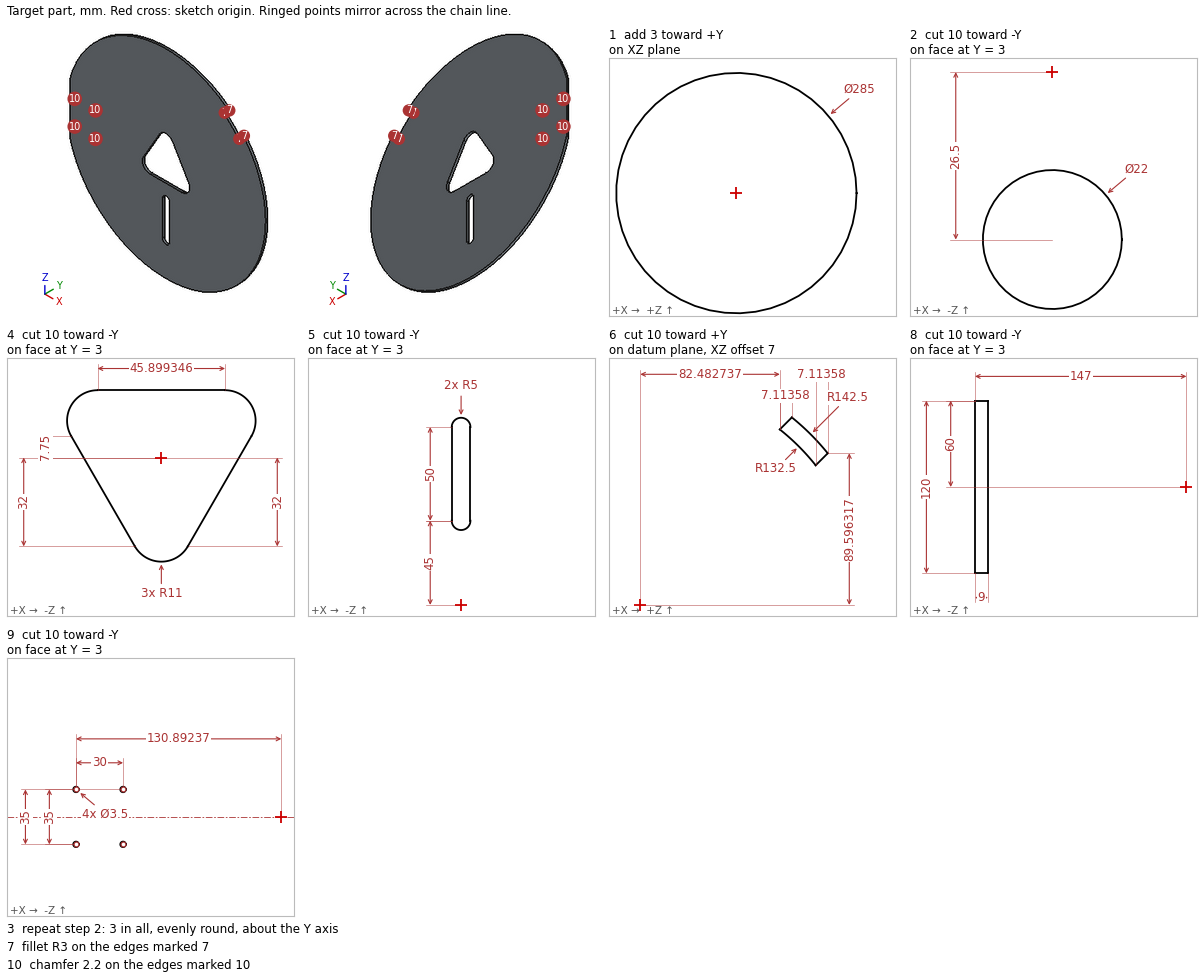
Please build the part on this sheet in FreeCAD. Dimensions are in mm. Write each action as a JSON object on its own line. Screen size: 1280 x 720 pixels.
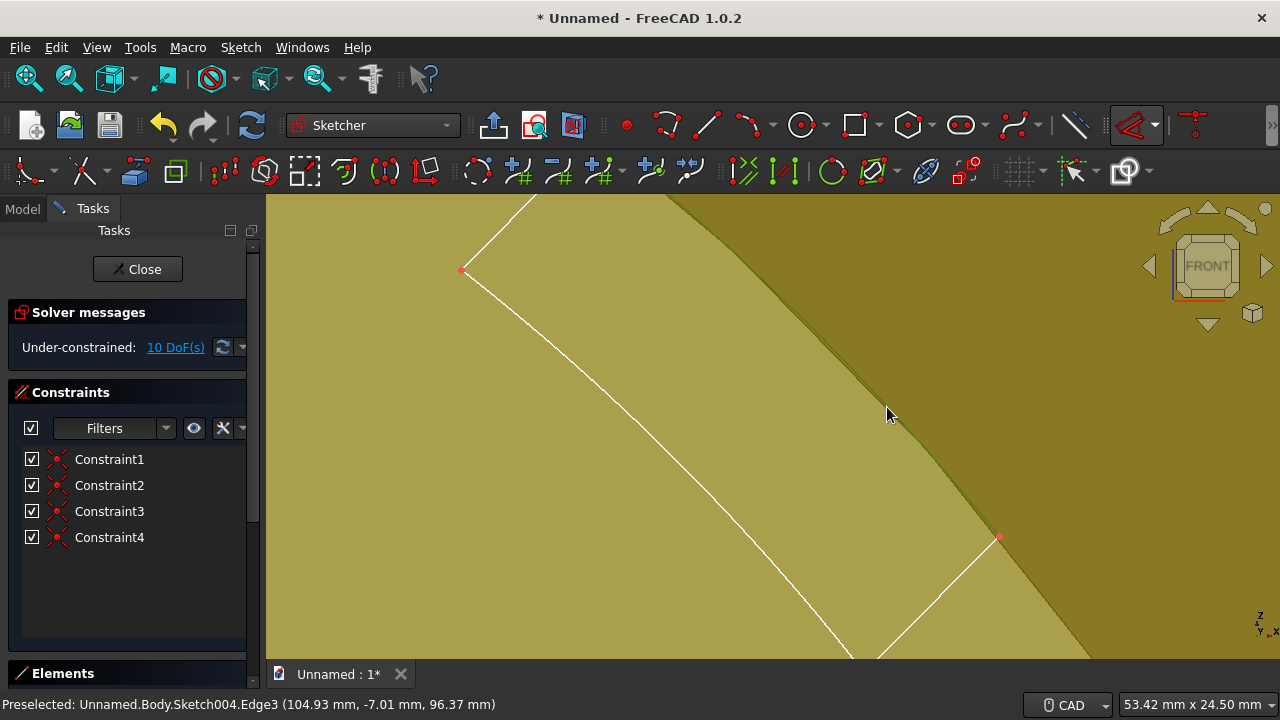
{"action": "left_click", "coordinate": [754, 542]}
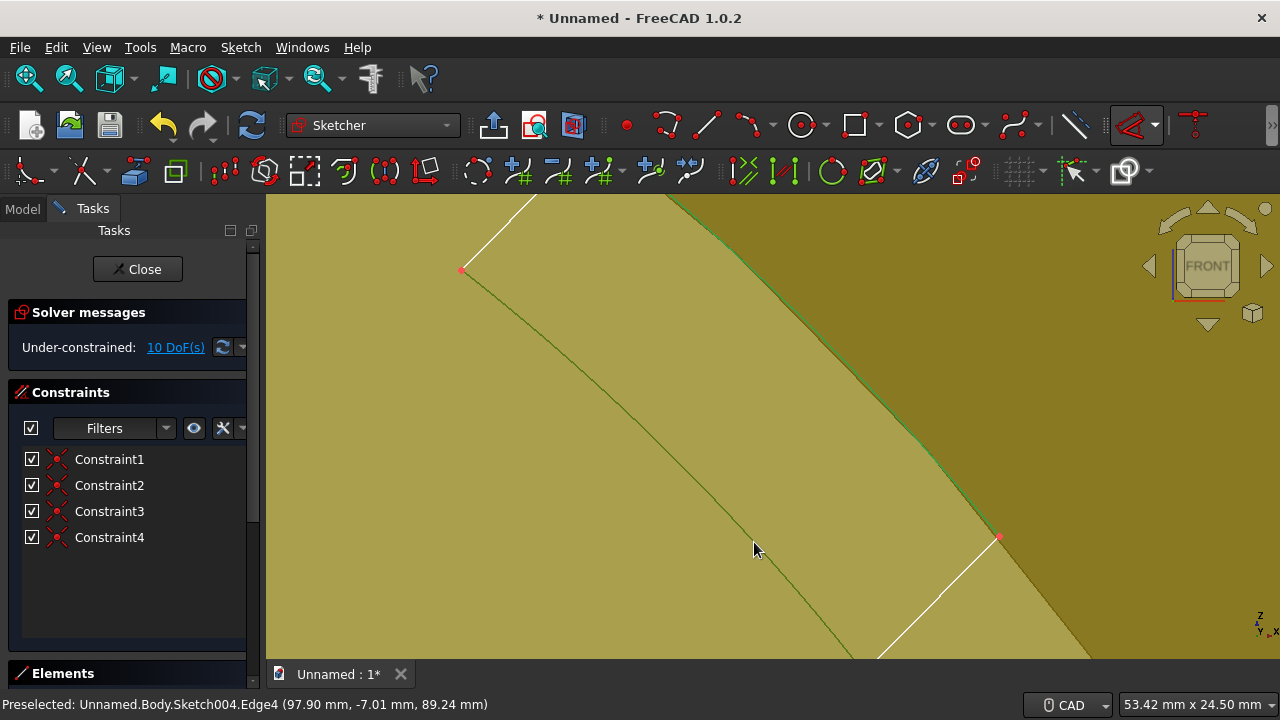
{"action": "left_click", "coordinate": [1194, 126]}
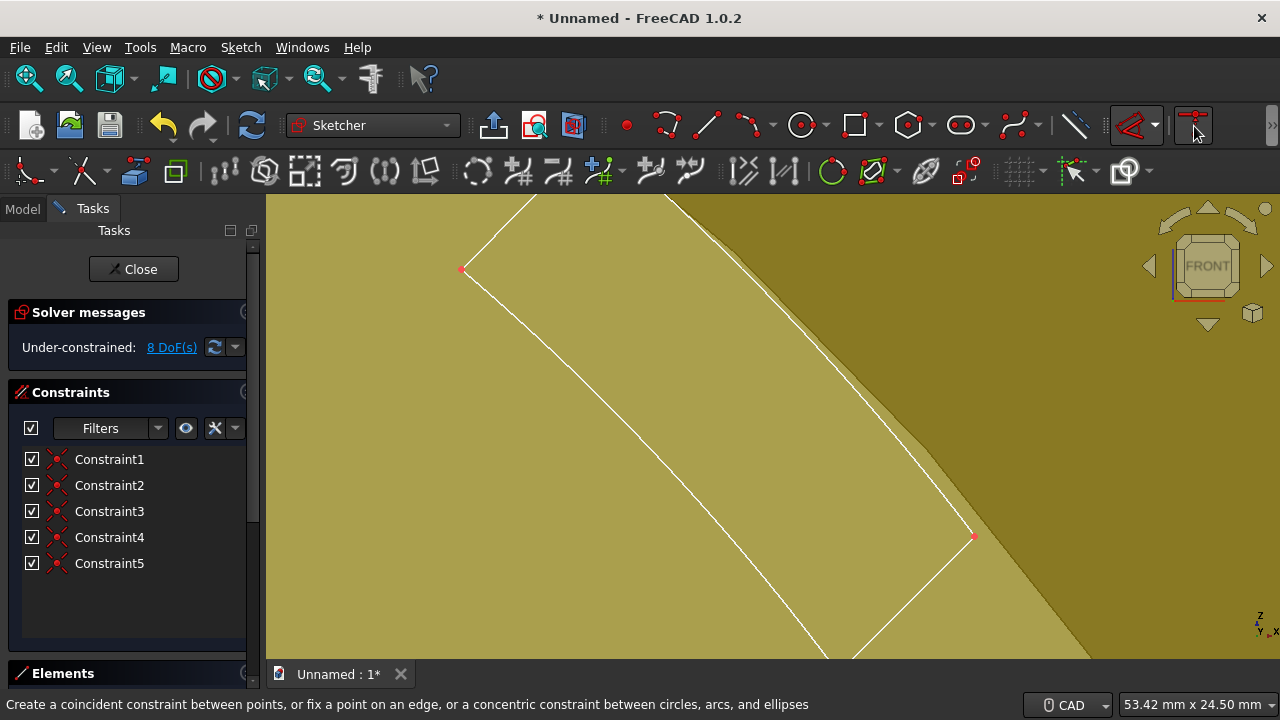
{"action": "scroll", "coordinate": [673, 457], "scroll_direction": "down", "scroll_amount": 3}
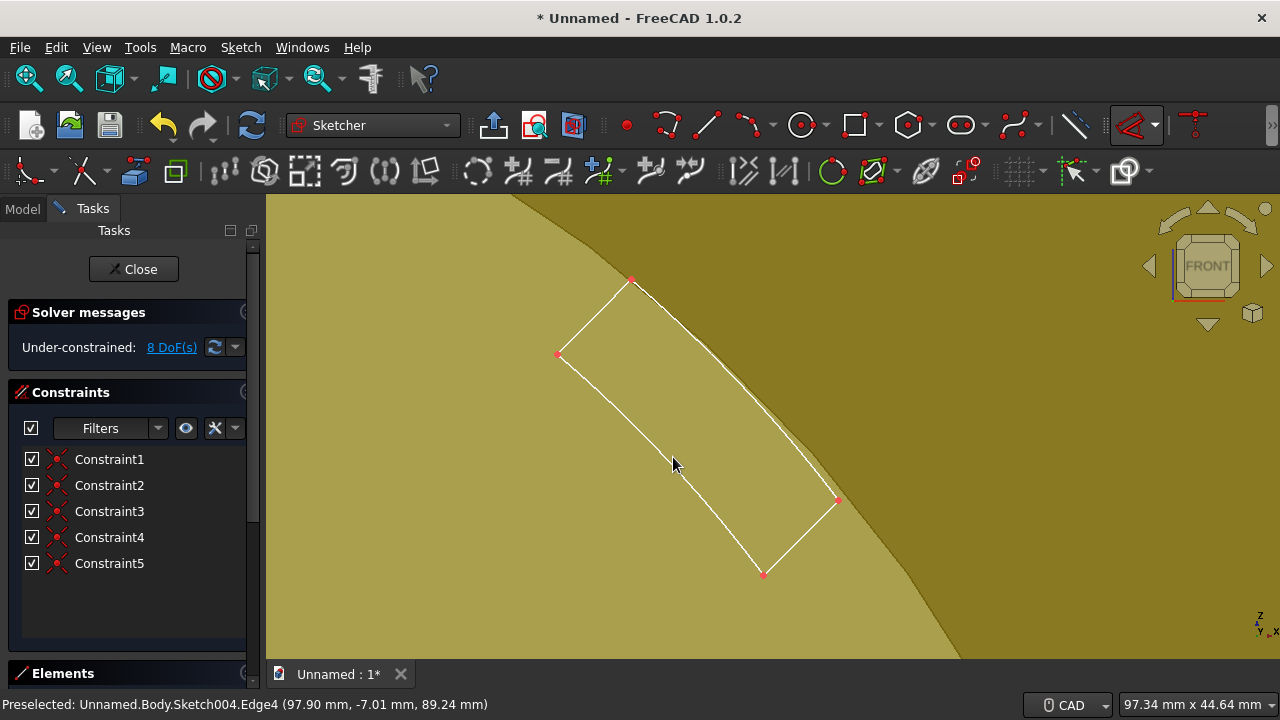
{"action": "scroll", "coordinate": [846, 291], "scroll_direction": "down", "scroll_amount": 7}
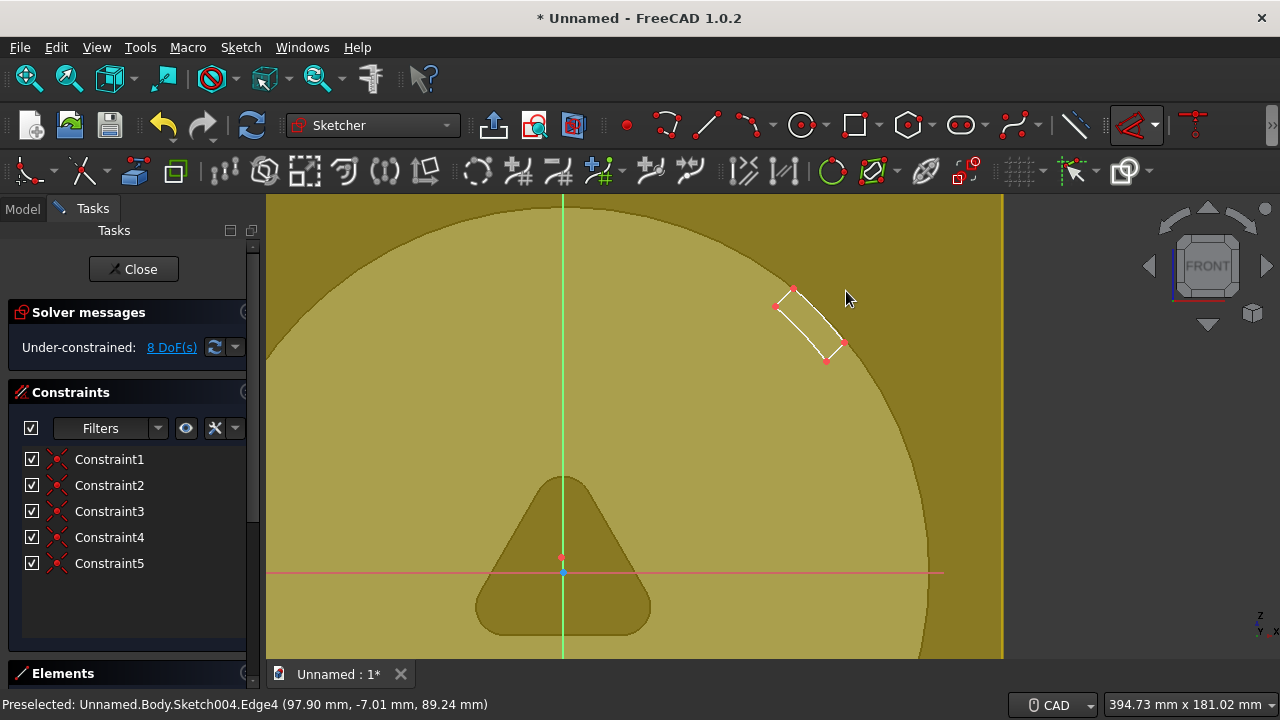
{"action": "left_click_drag", "start_coordinate": [552, 548], "coordinate": [573, 583]}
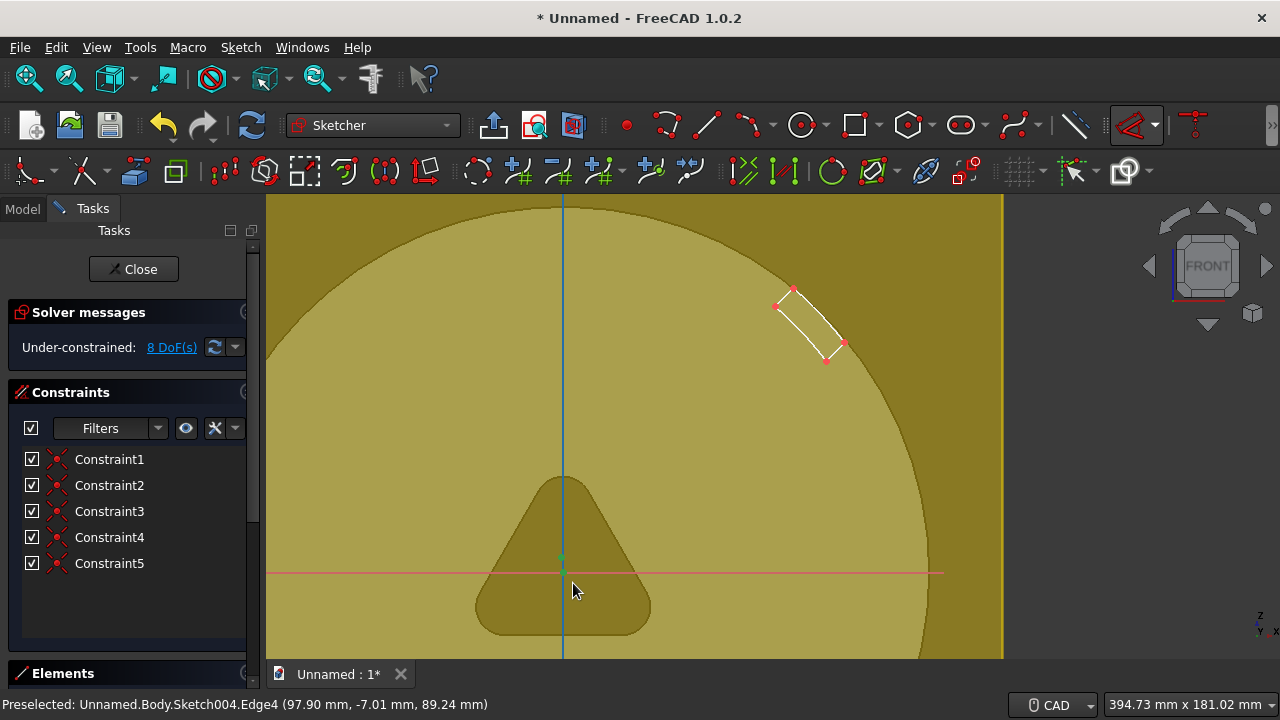
{"action": "left_click", "coordinate": [1194, 126]}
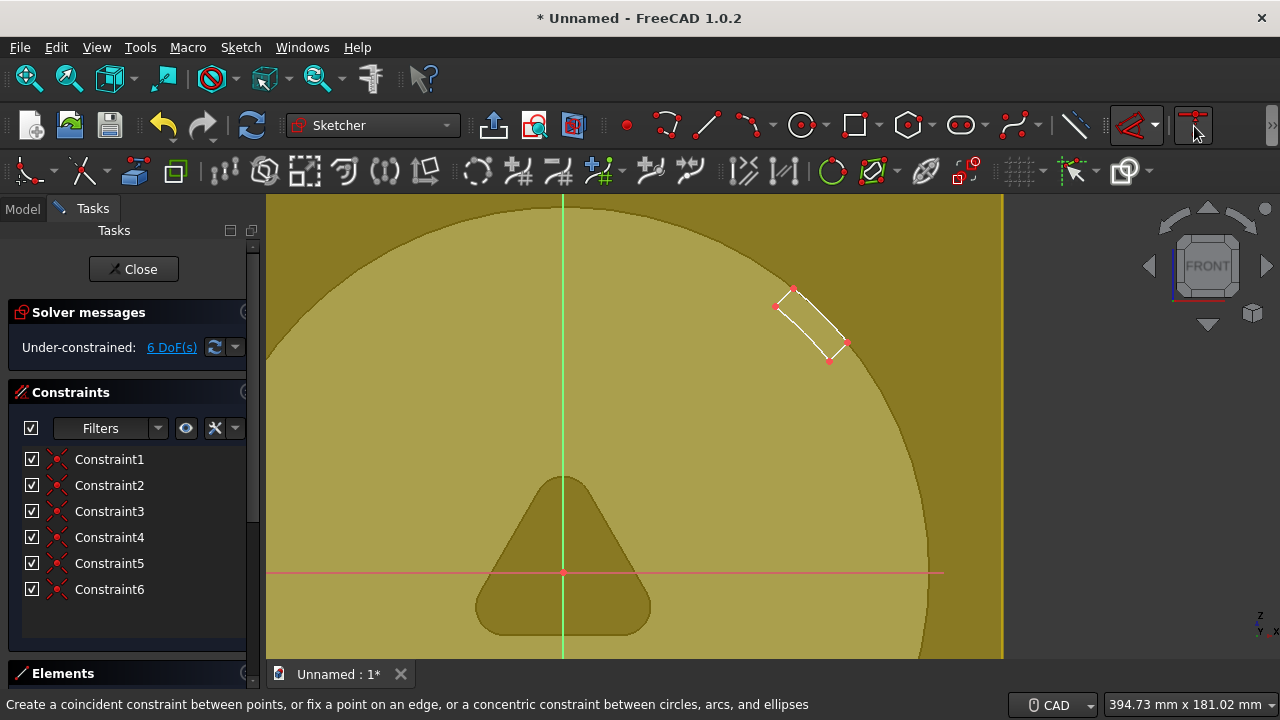
{"action": "left_click", "coordinate": [833, 325]}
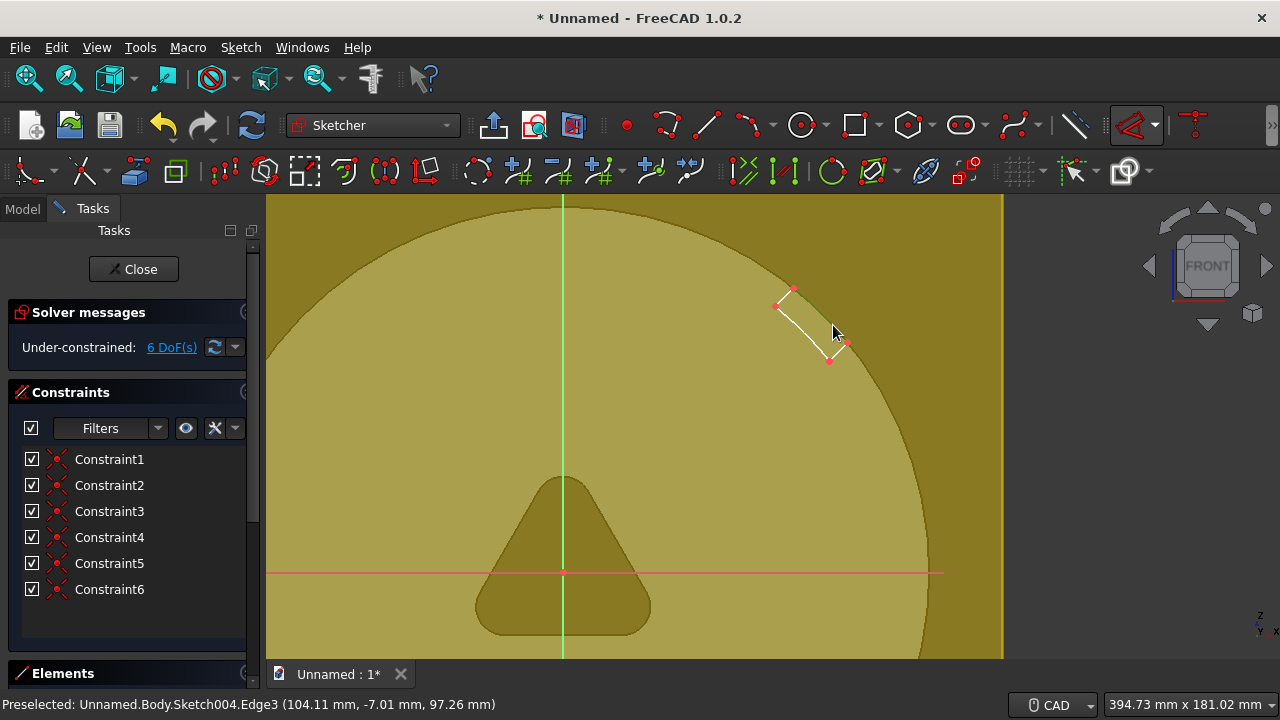
{"action": "left_click", "coordinate": [1158, 126]}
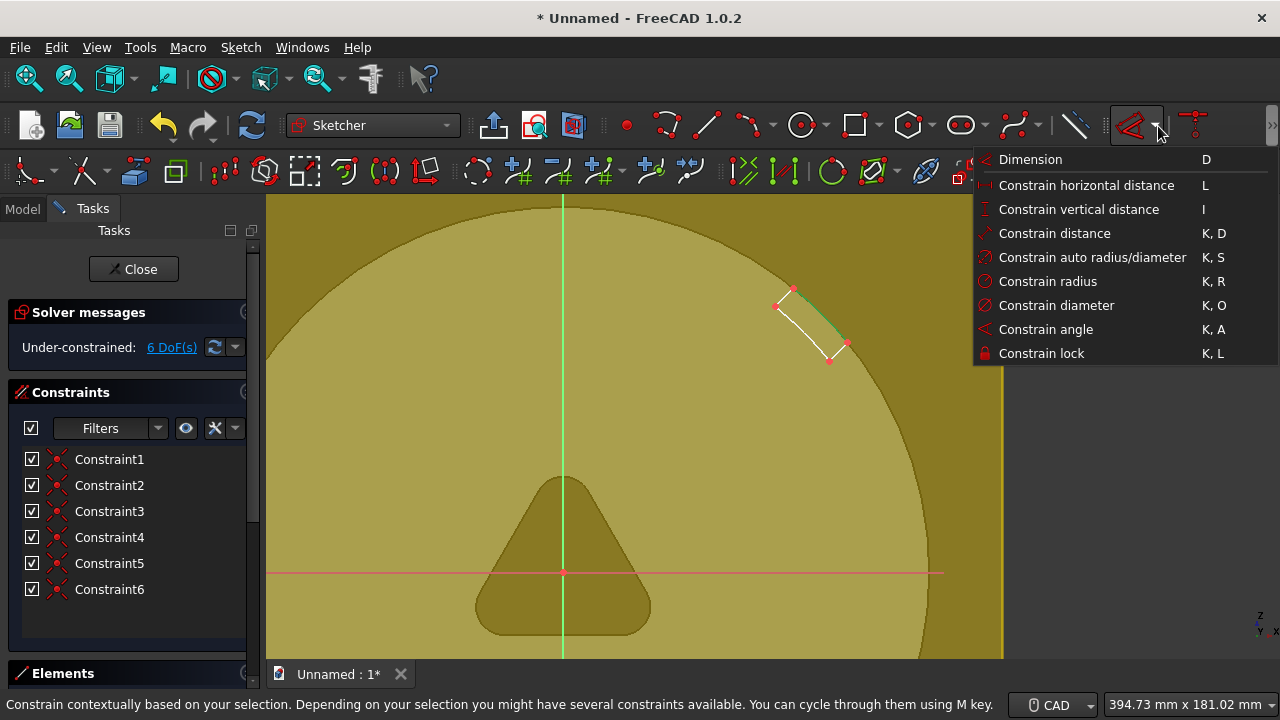
{"action": "left_click", "coordinate": [1126, 281]}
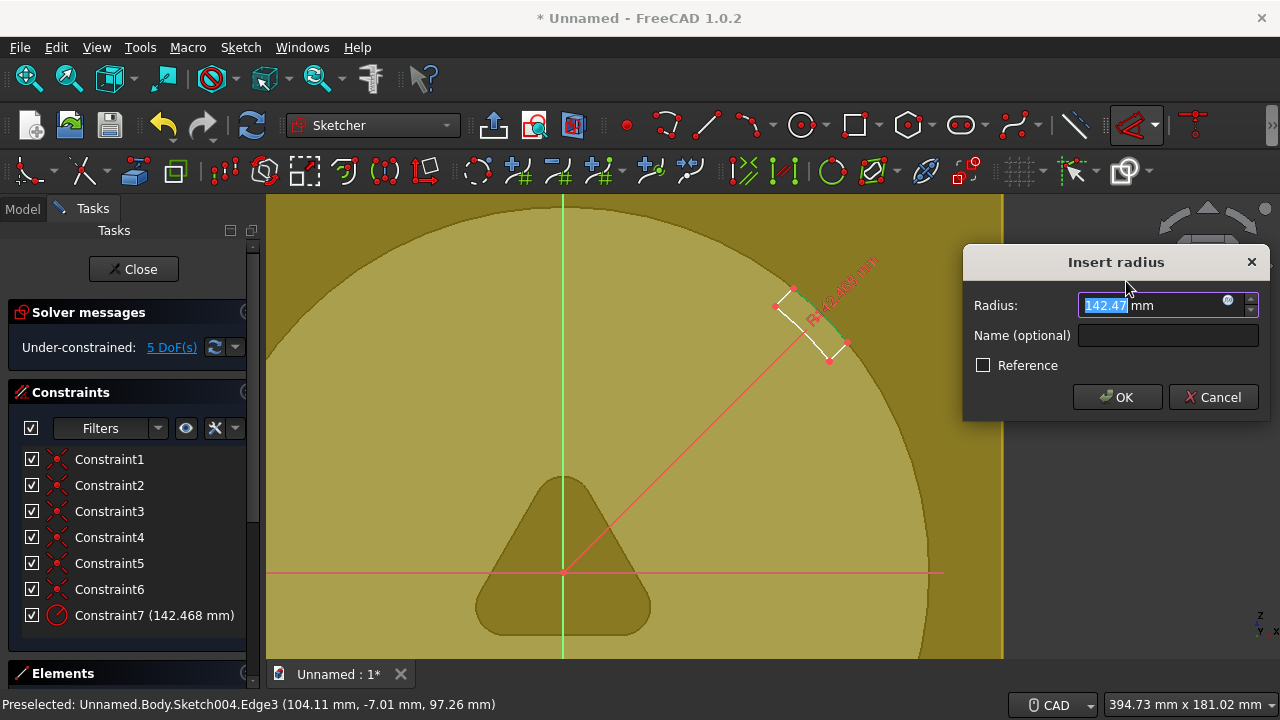
{"action": "type", "text": "142.5"}
{"action": "key", "text": "Return"}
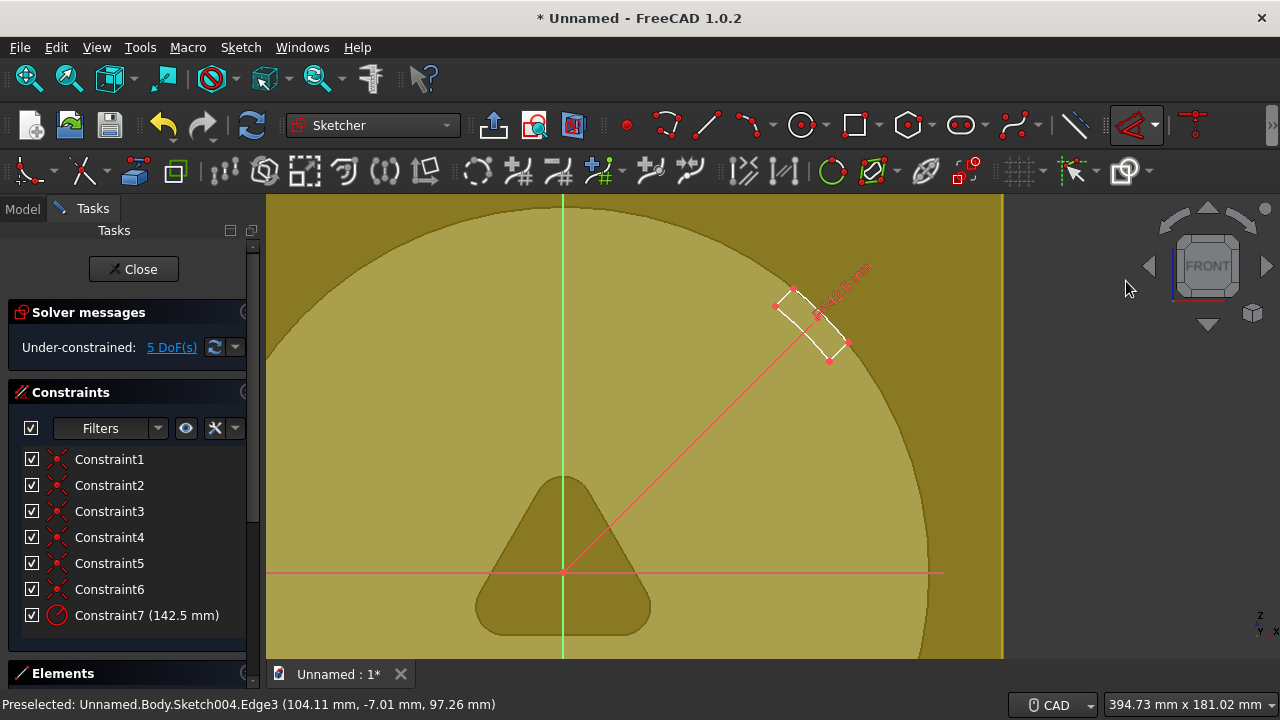
{"action": "left_click", "coordinate": [815, 344]}